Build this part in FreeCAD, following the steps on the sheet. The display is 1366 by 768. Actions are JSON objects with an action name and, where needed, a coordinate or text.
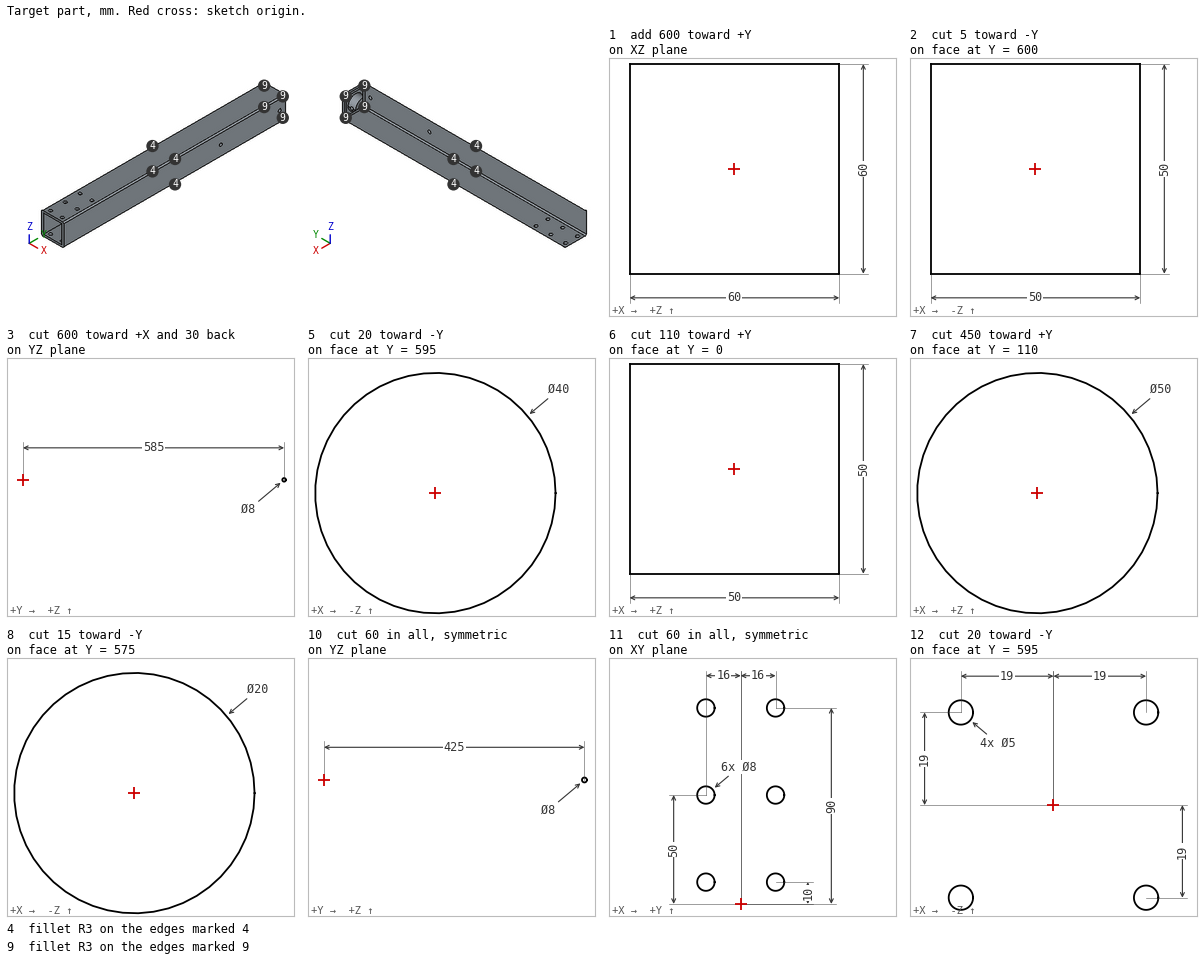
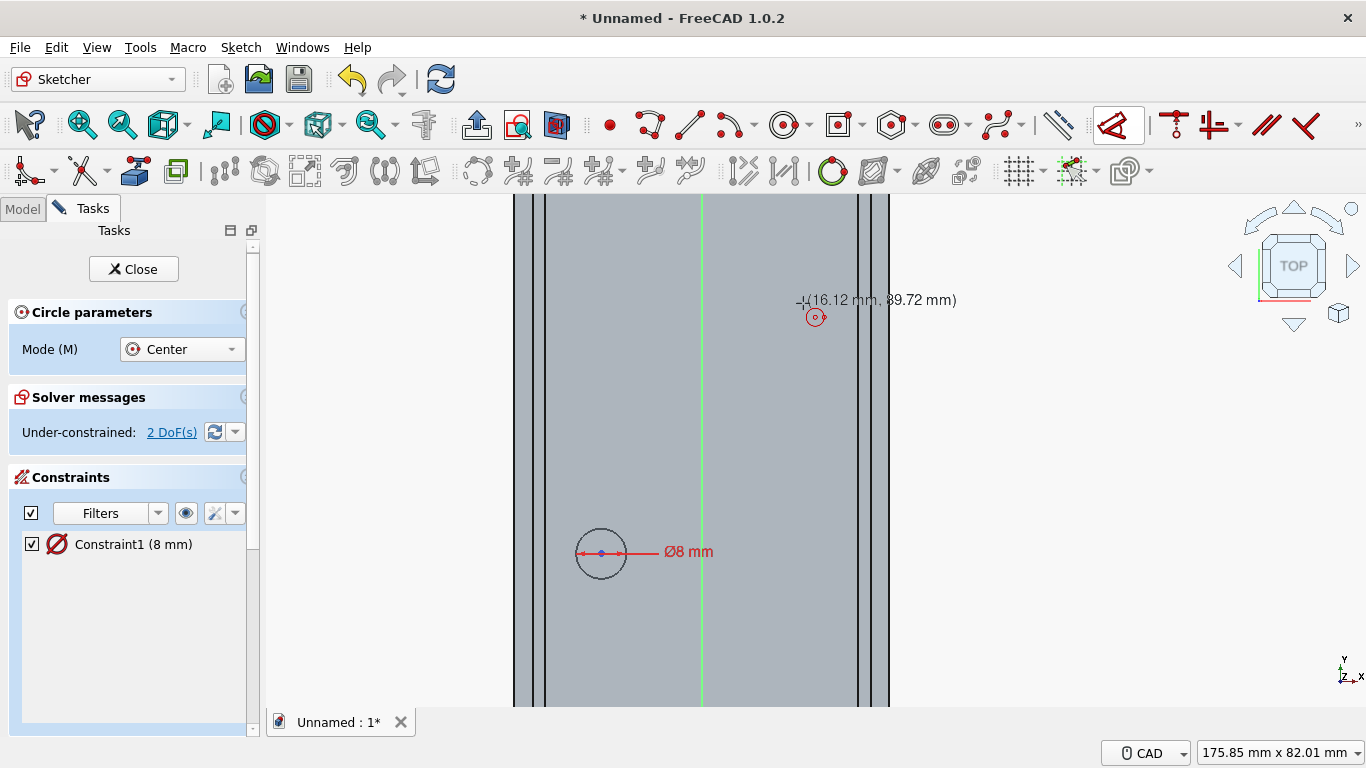
{"action": "left_click", "coordinate": [802, 303]}
{"action": "mouse_move", "coordinate": [820, 285]}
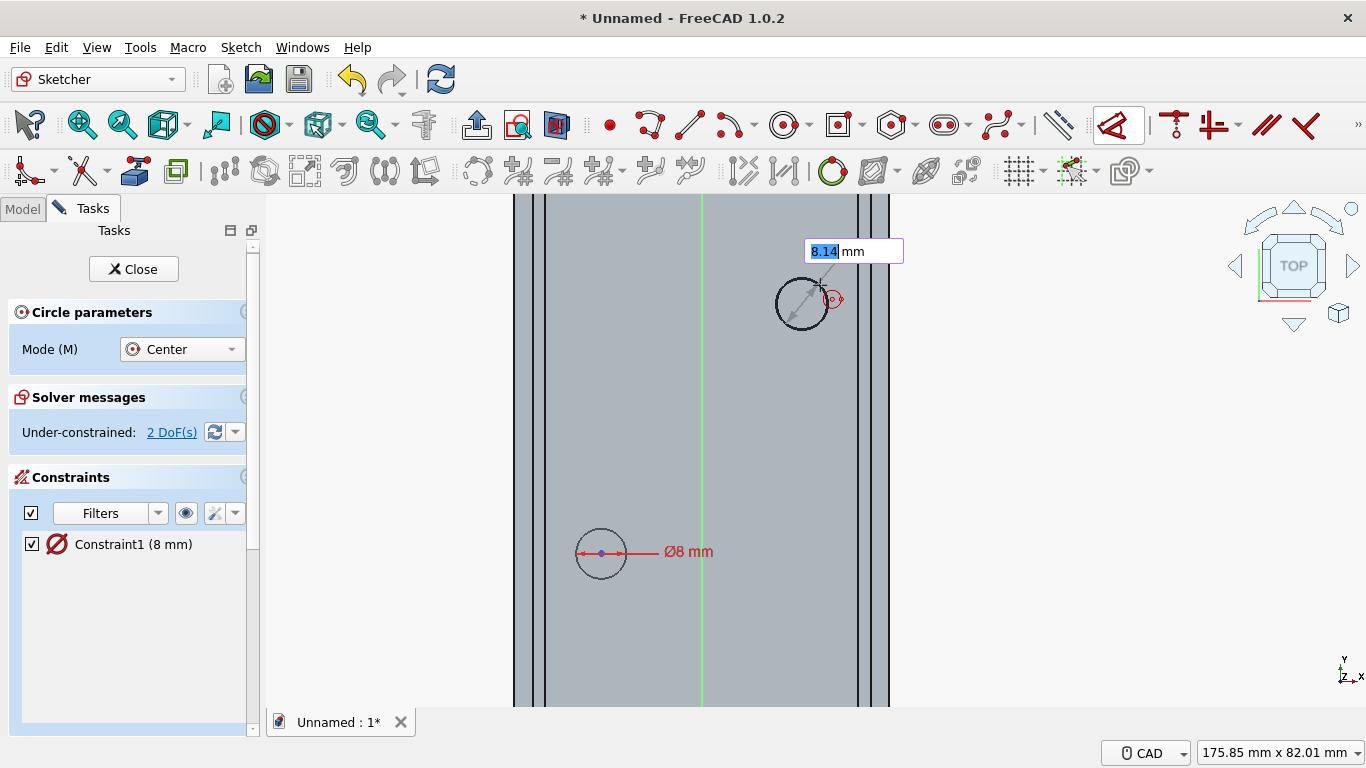
{"action": "type", "text": "8"}
{"action": "key", "text": "Return"}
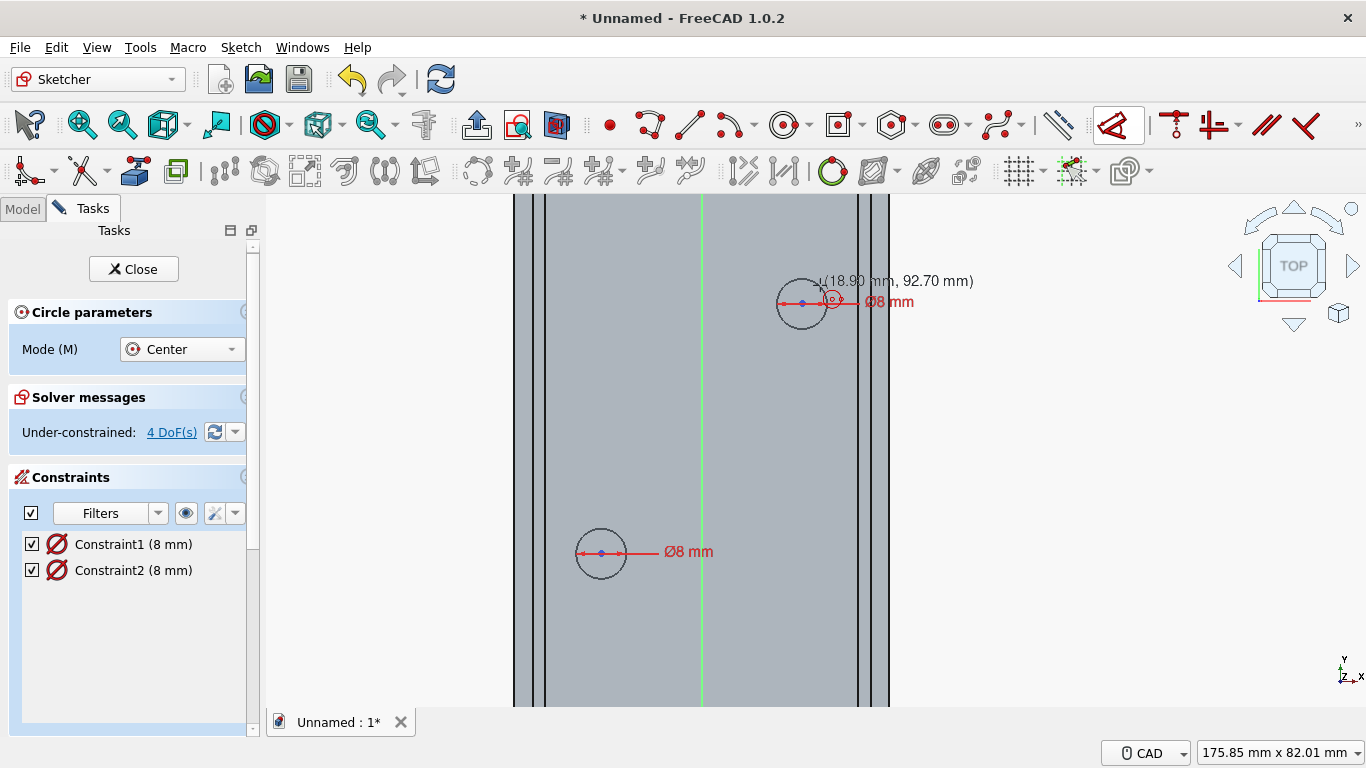
{"action": "left_click", "coordinate": [802, 553]}
{"action": "mouse_move", "coordinate": [820, 535]}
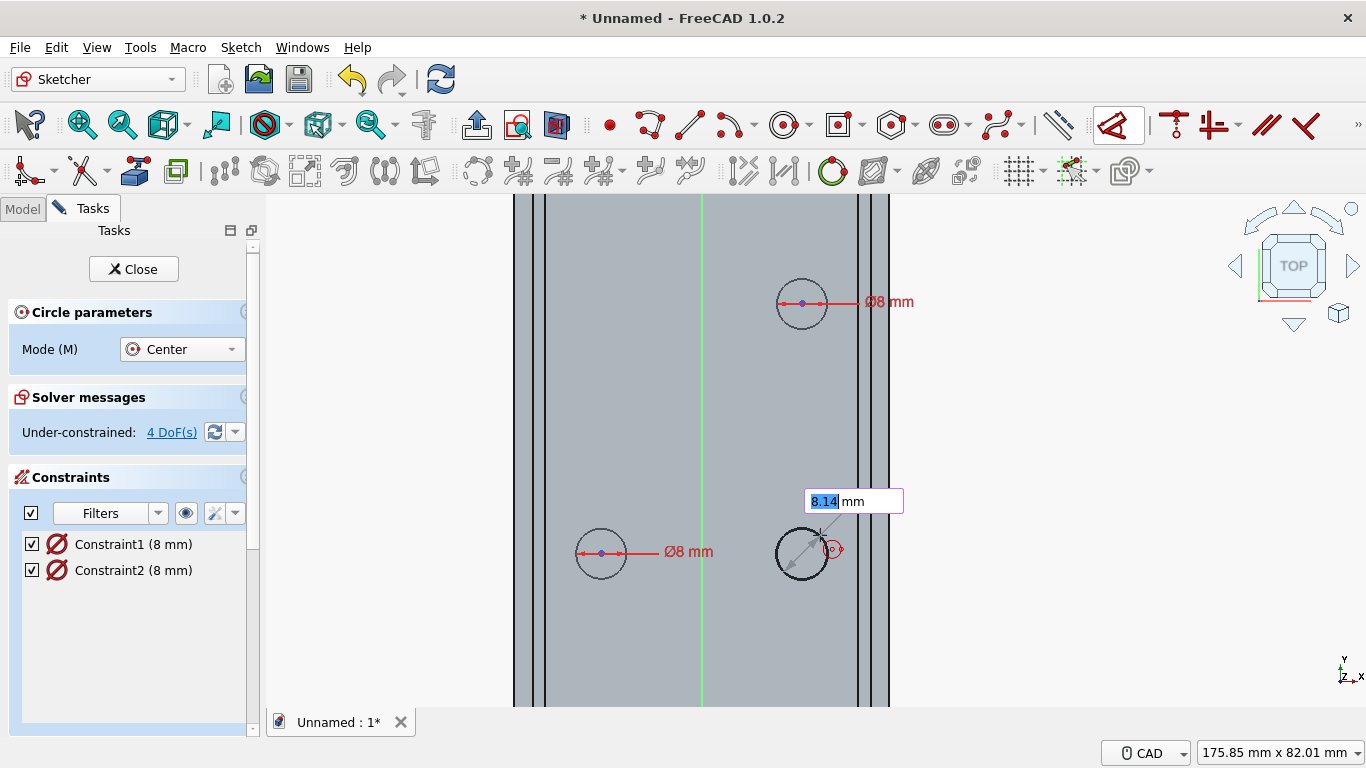
{"action": "type", "text": "8"}
{"action": "key", "text": "Return"}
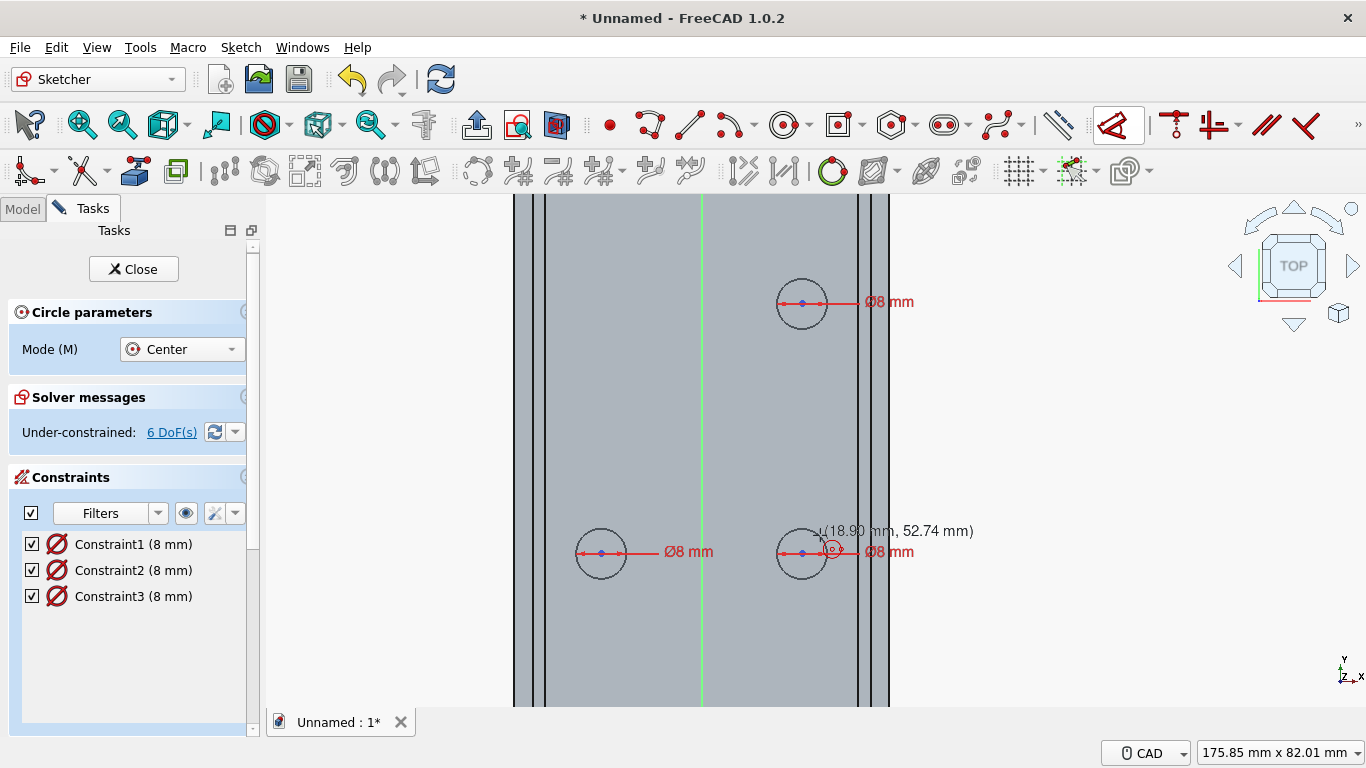
{"action": "left_click", "coordinate": [602, 303]}
{"action": "mouse_move", "coordinate": [619, 285]}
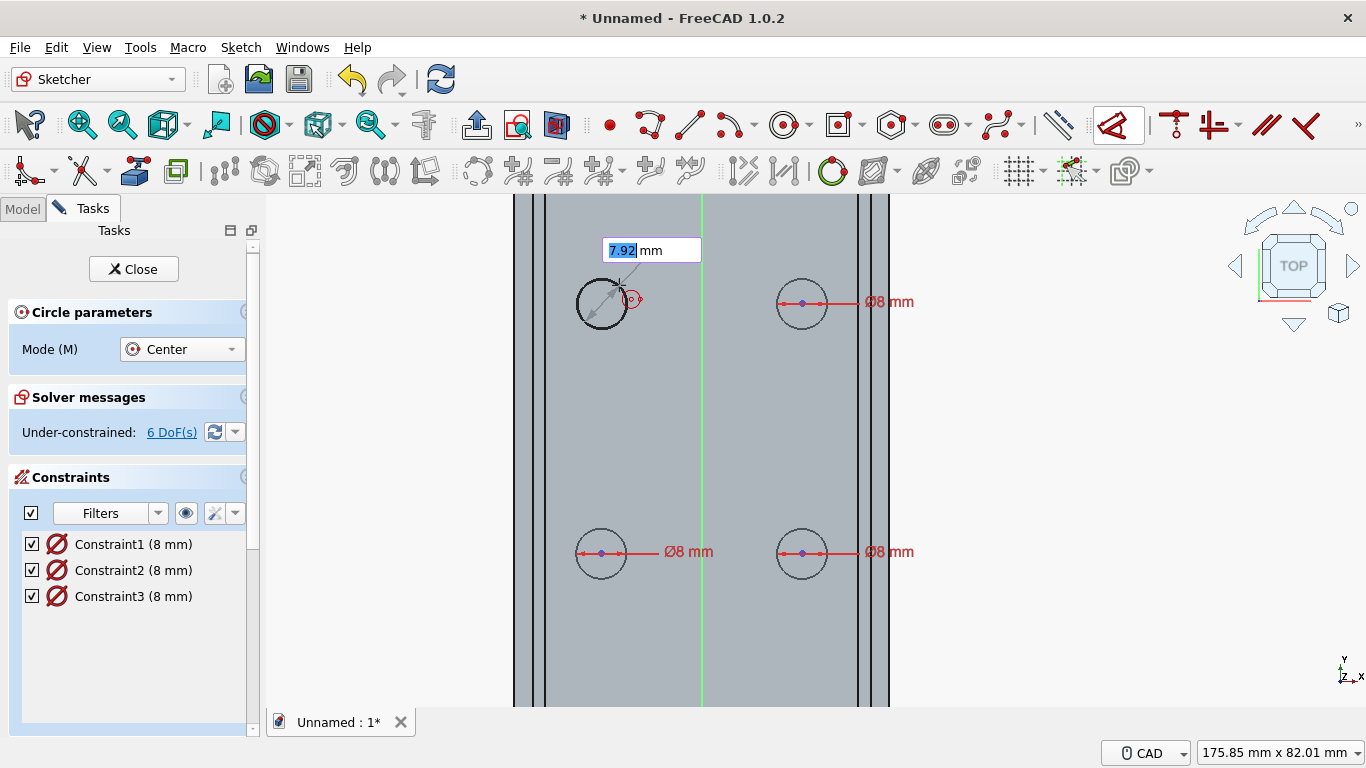
{"action": "type", "text": "8"}
{"action": "key", "text": "Return"}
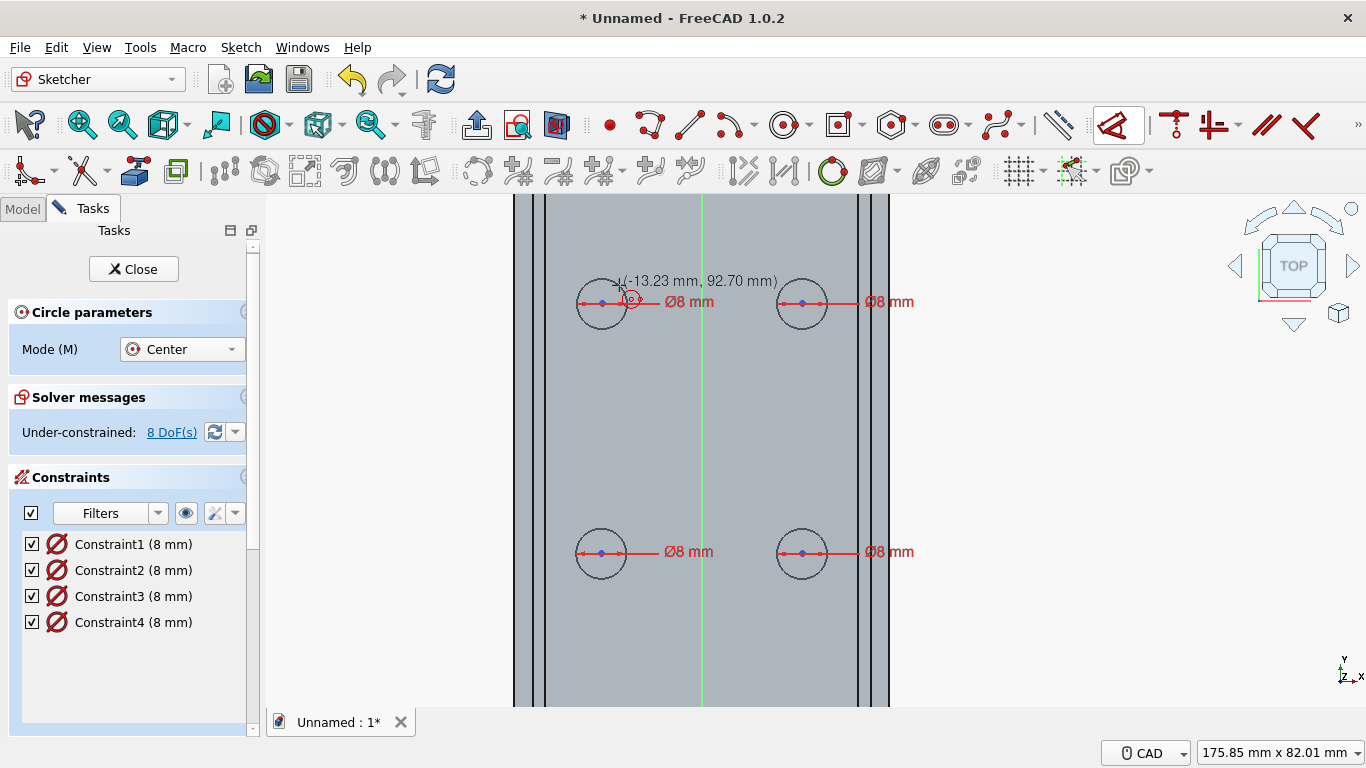
{"action": "scroll", "coordinate": [803, 303], "scroll_direction": "down", "scroll_amount": 3}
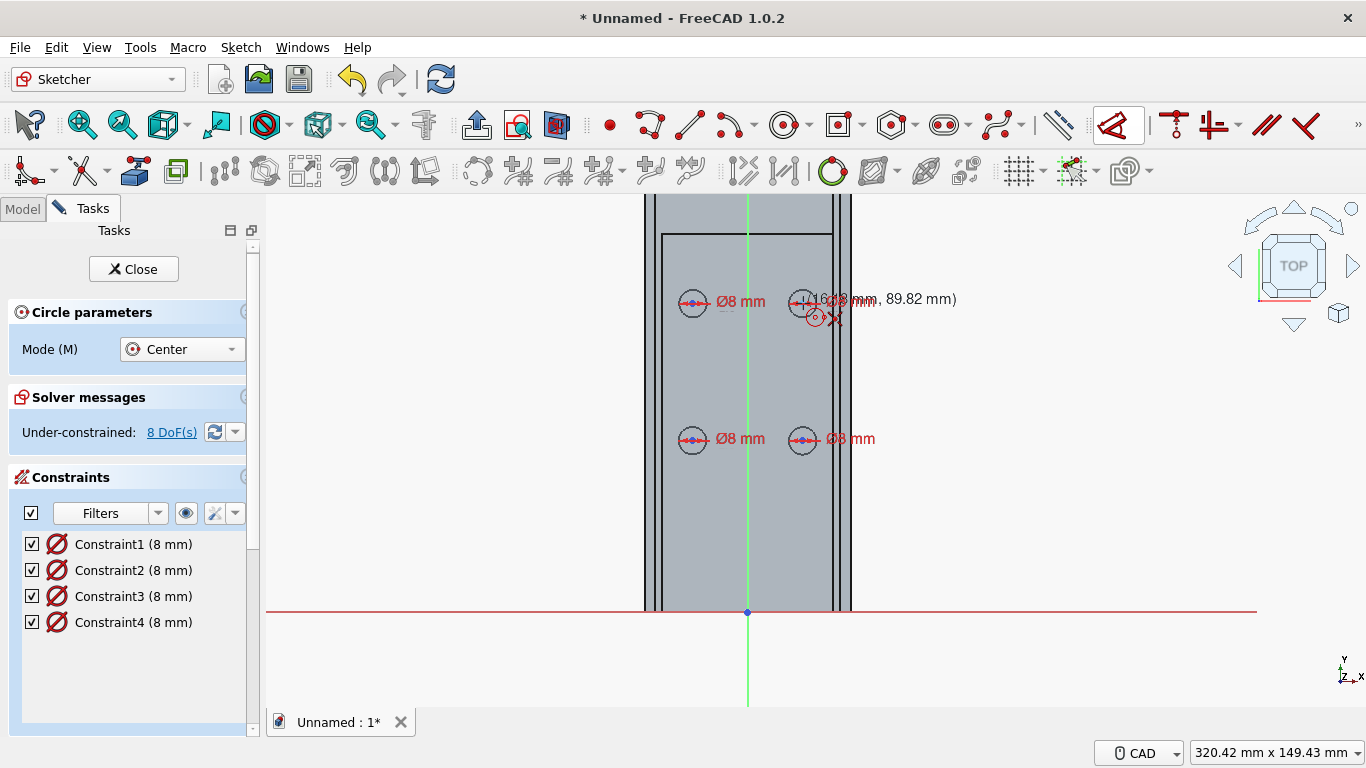
{"action": "scroll", "coordinate": [803, 578], "scroll_direction": "up", "scroll_amount": 3}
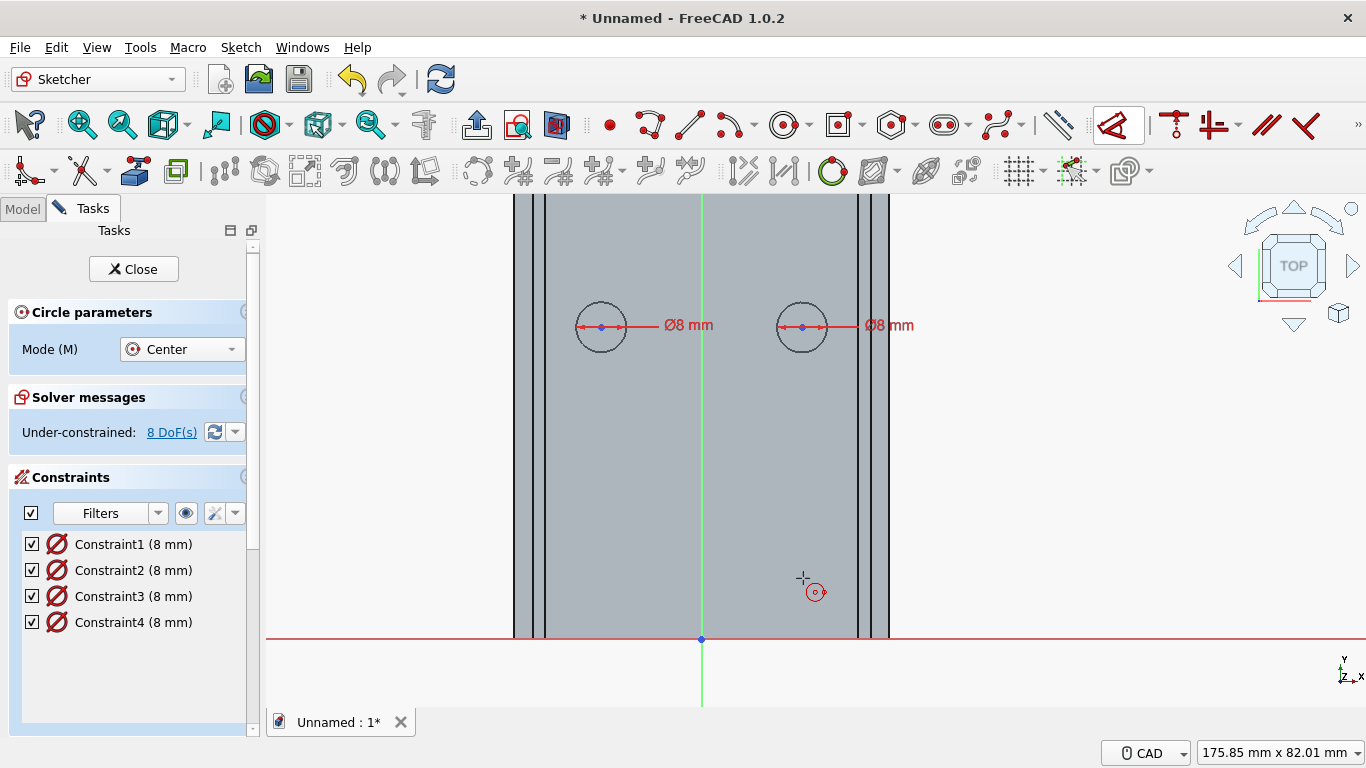
{"action": "left_click", "coordinate": [802, 577]}
{"action": "mouse_move", "coordinate": [820, 559]}